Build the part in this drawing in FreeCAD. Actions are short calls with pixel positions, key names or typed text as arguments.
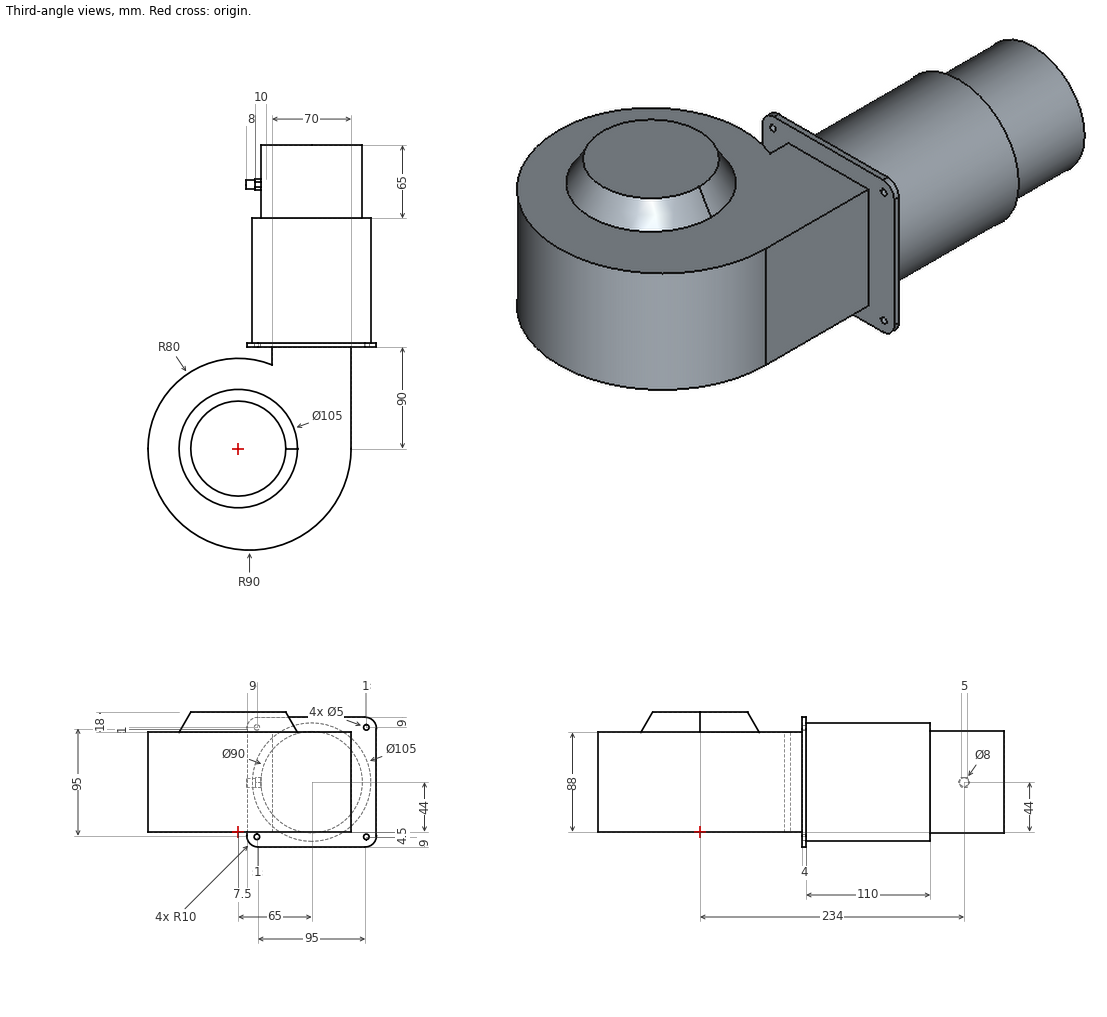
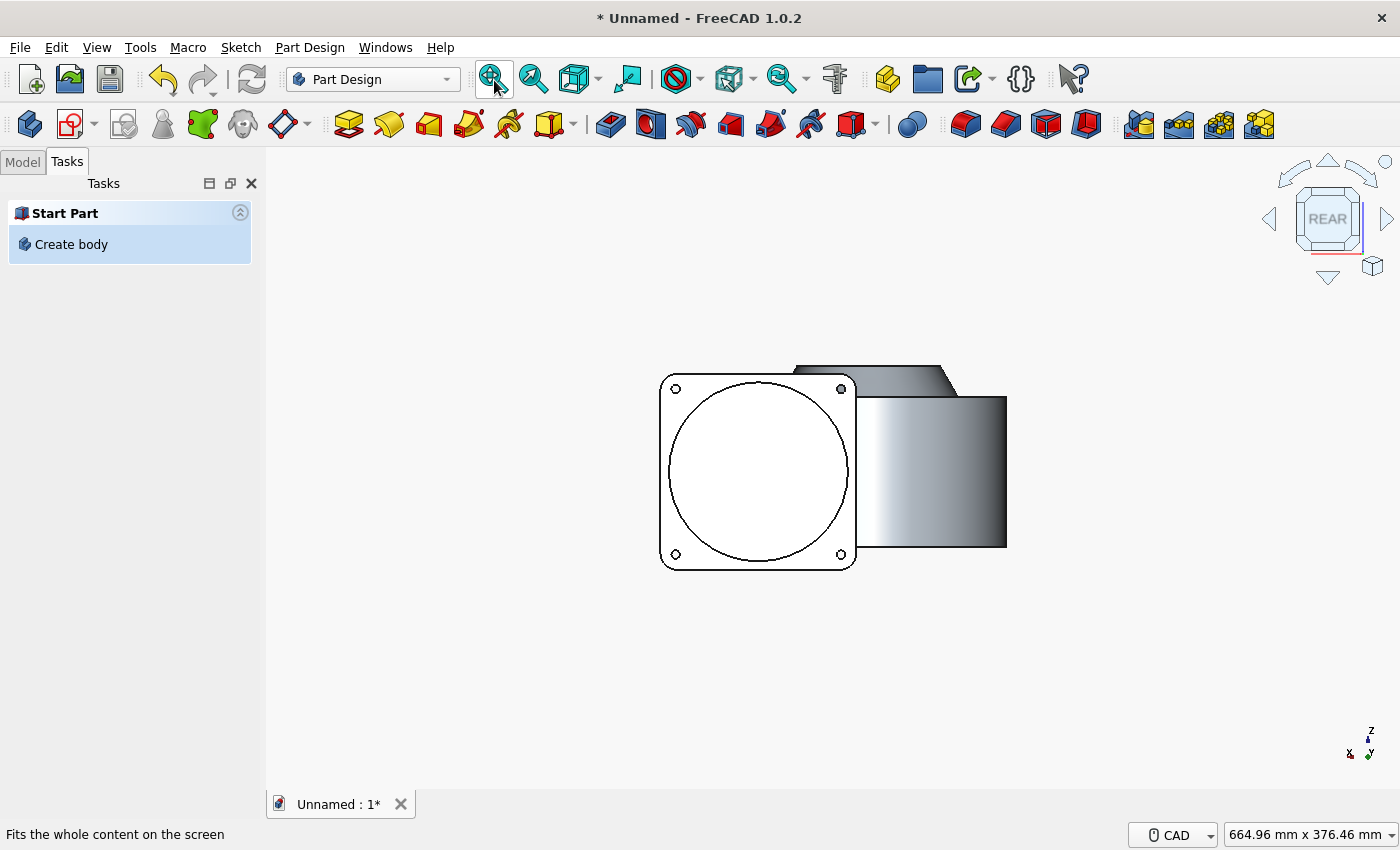
click(758, 471)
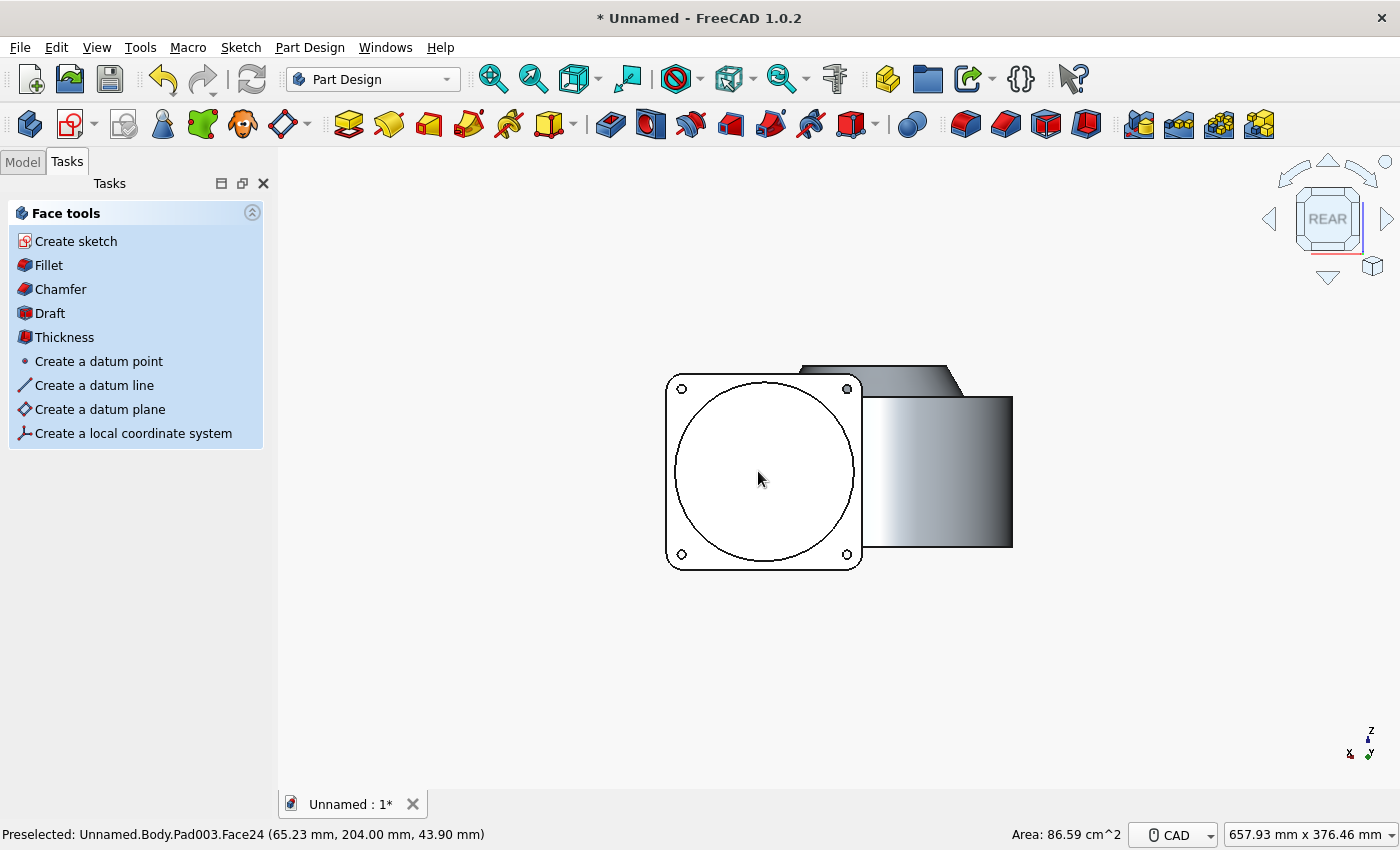
click(70, 124)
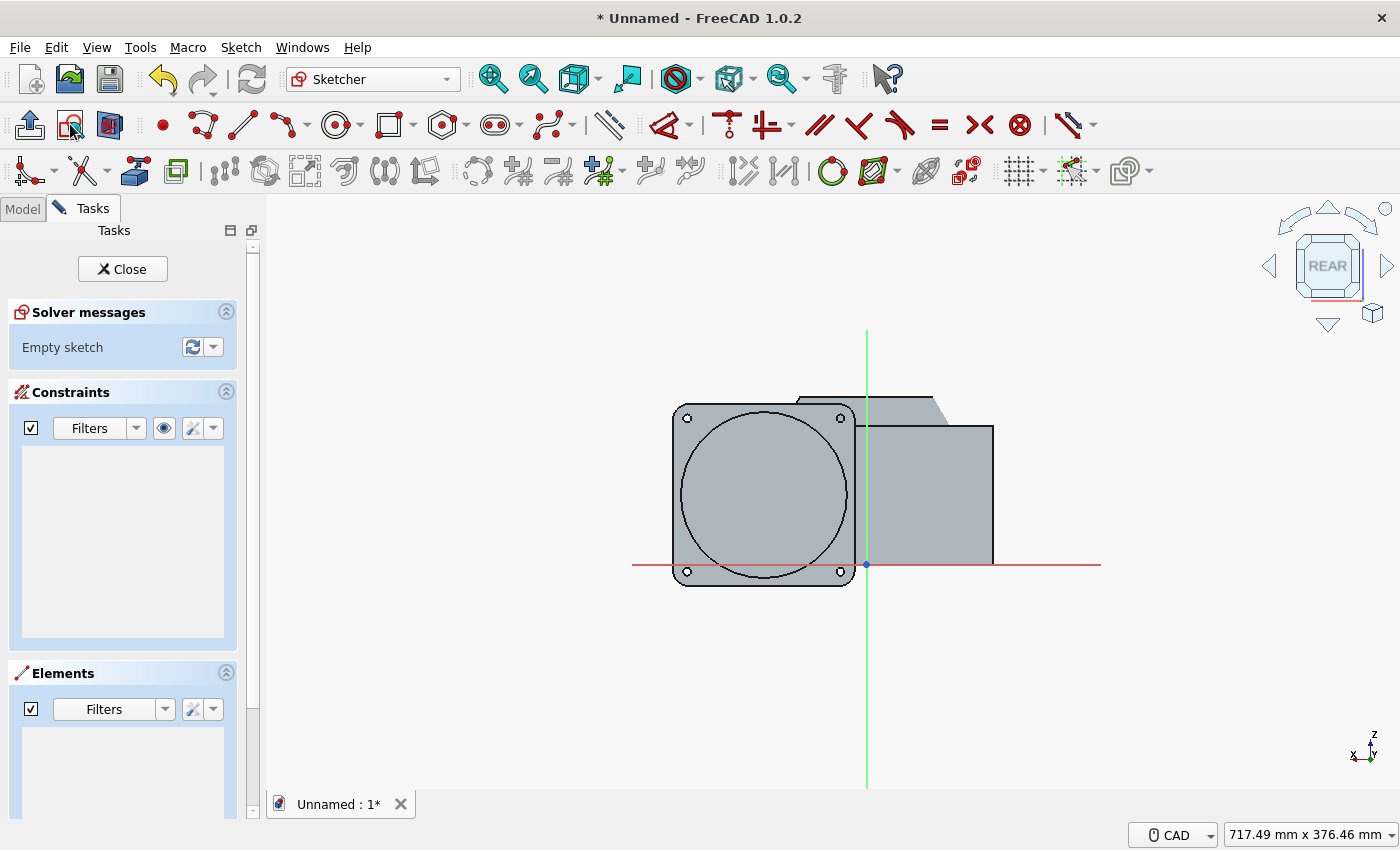
scroll(788, 497, up, 5)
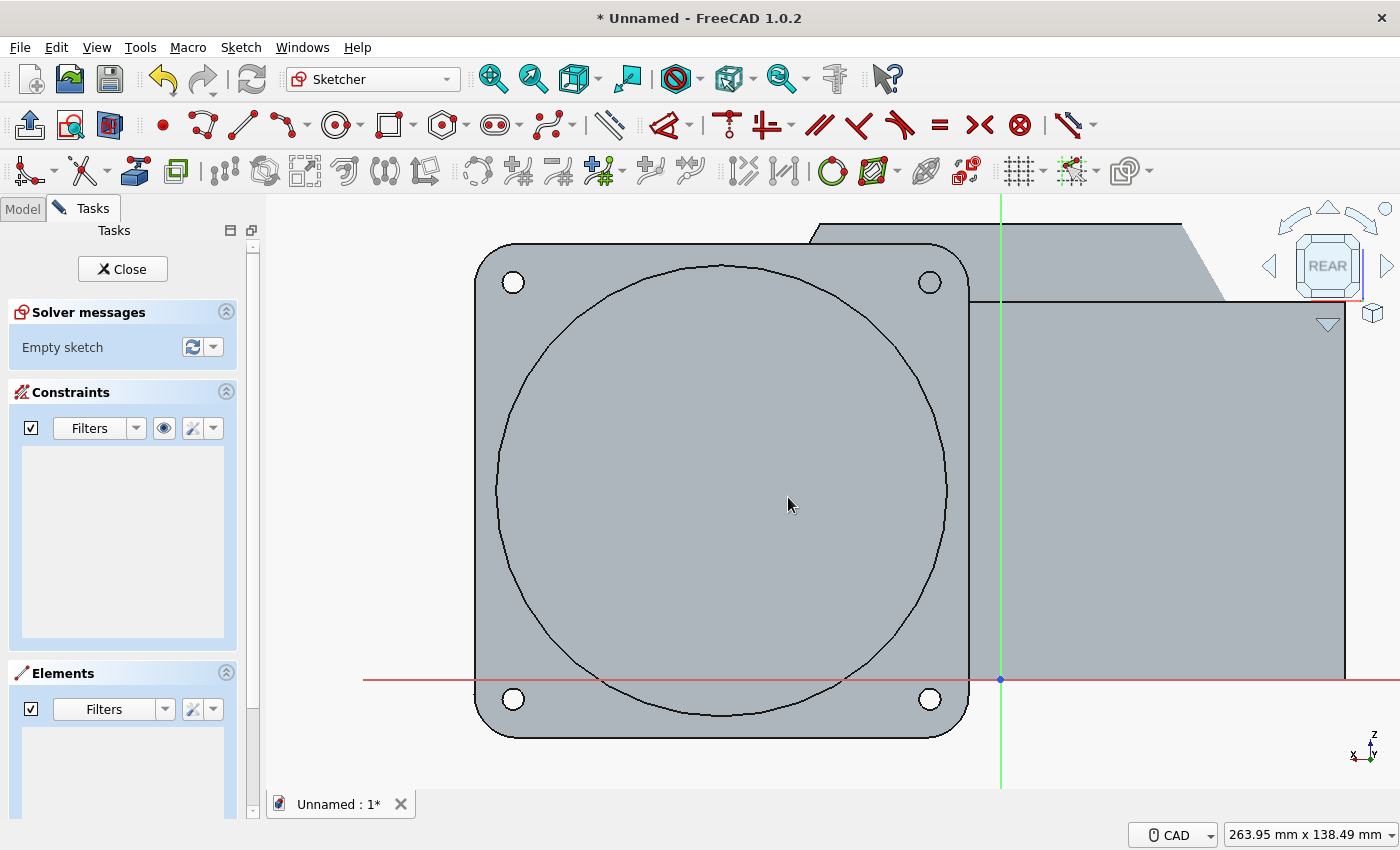
click(336, 126)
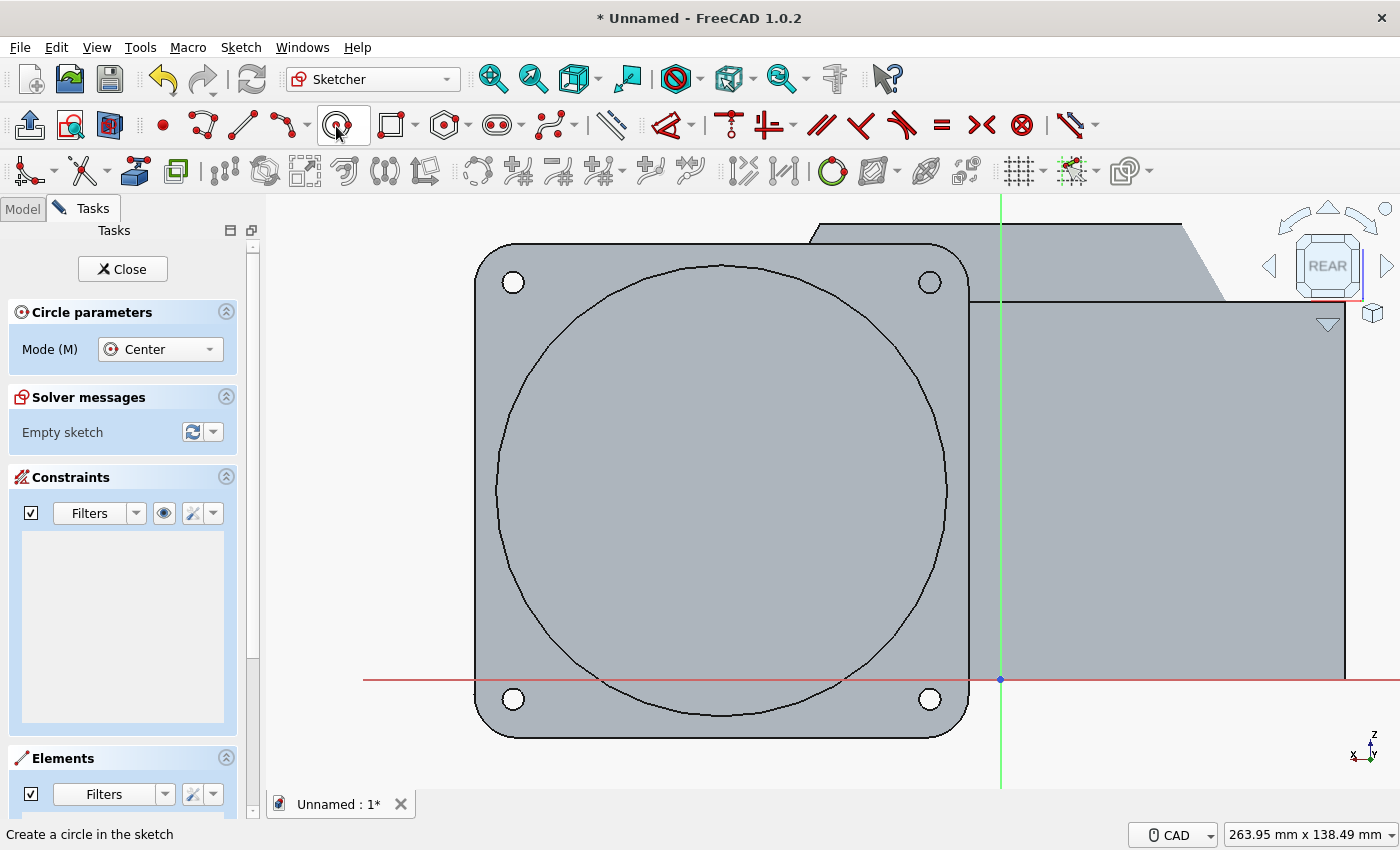
click(722, 491)
click(858, 354)
key(Escape)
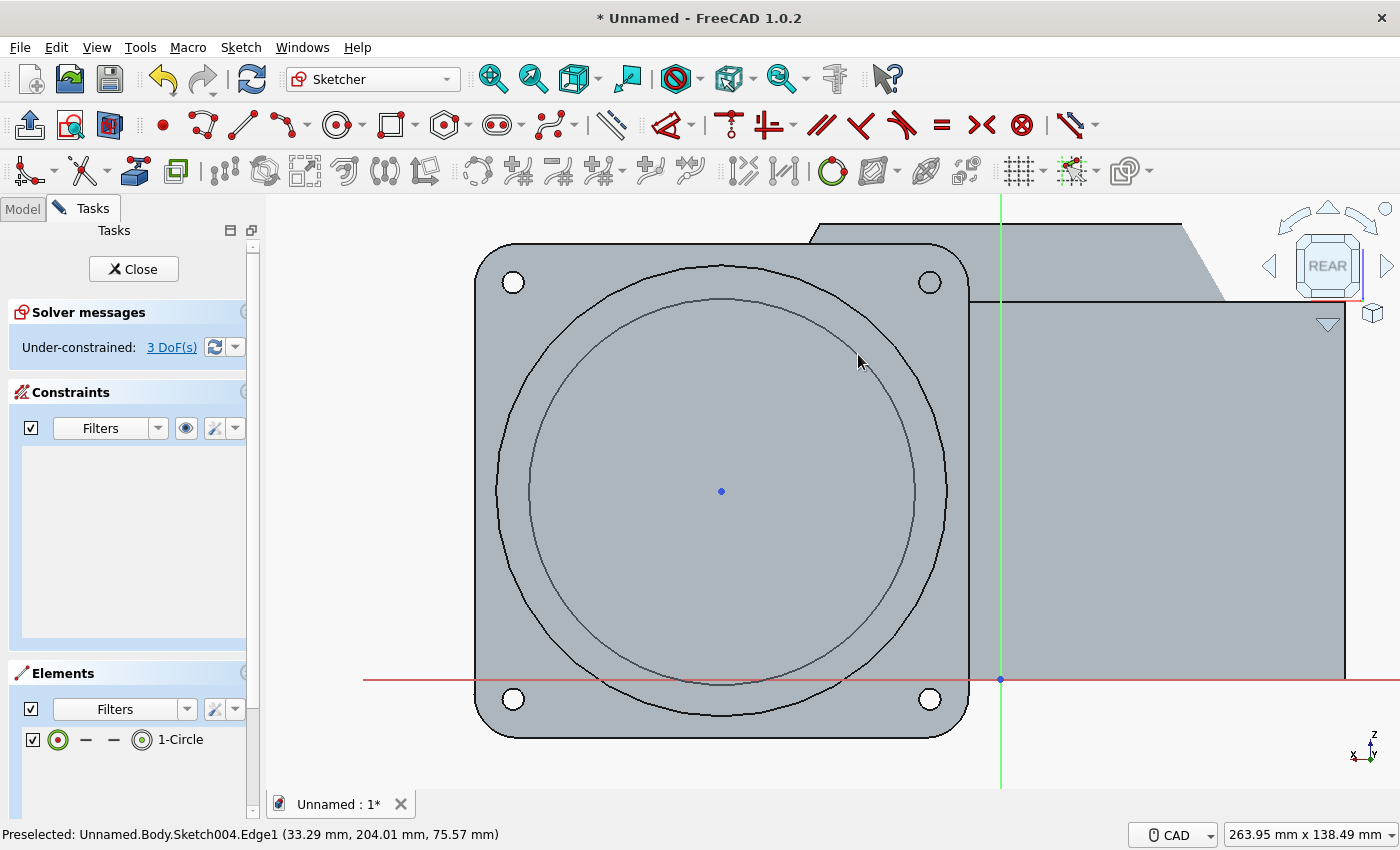
click(666, 126)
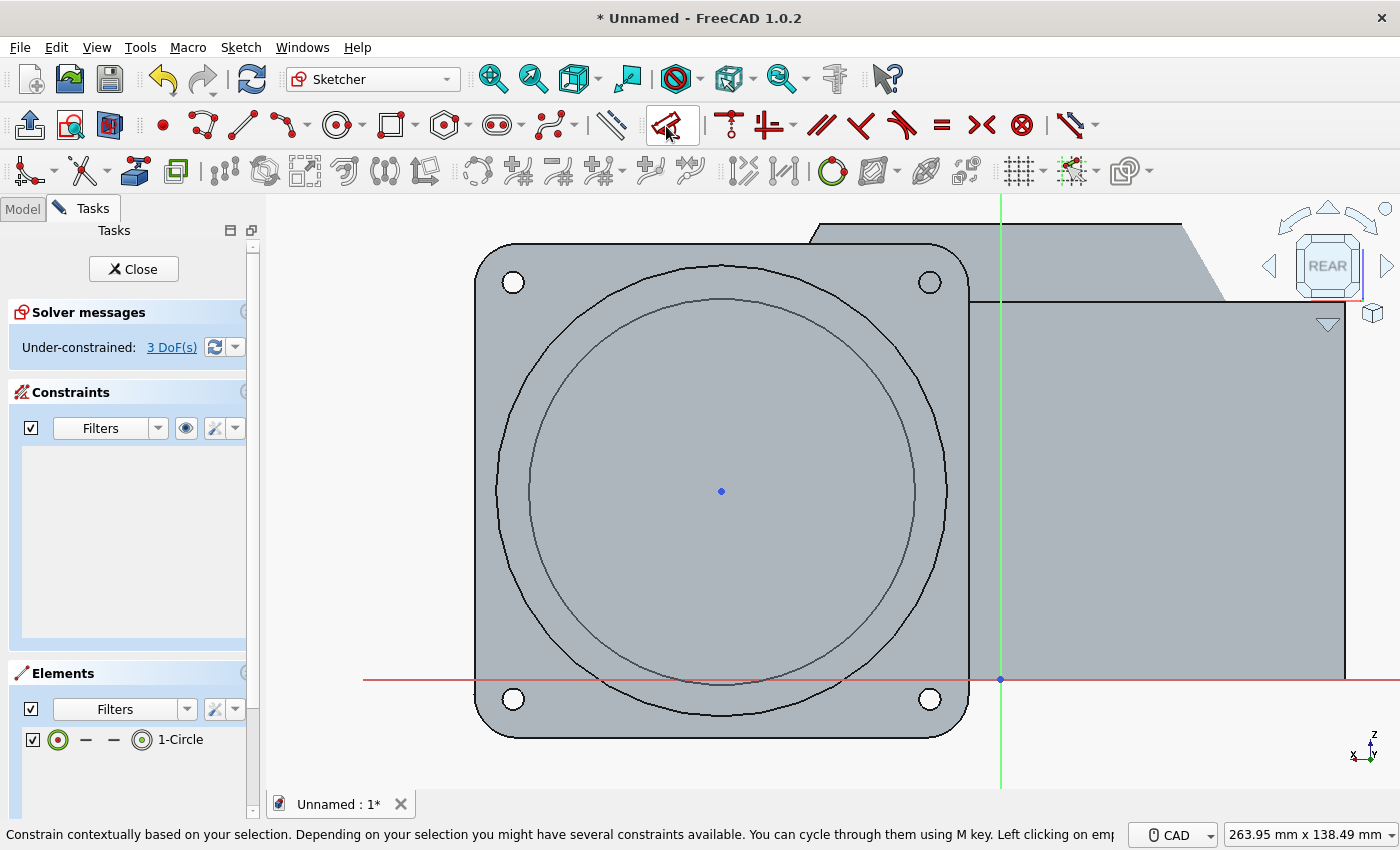
click(858, 355)
click(881, 332)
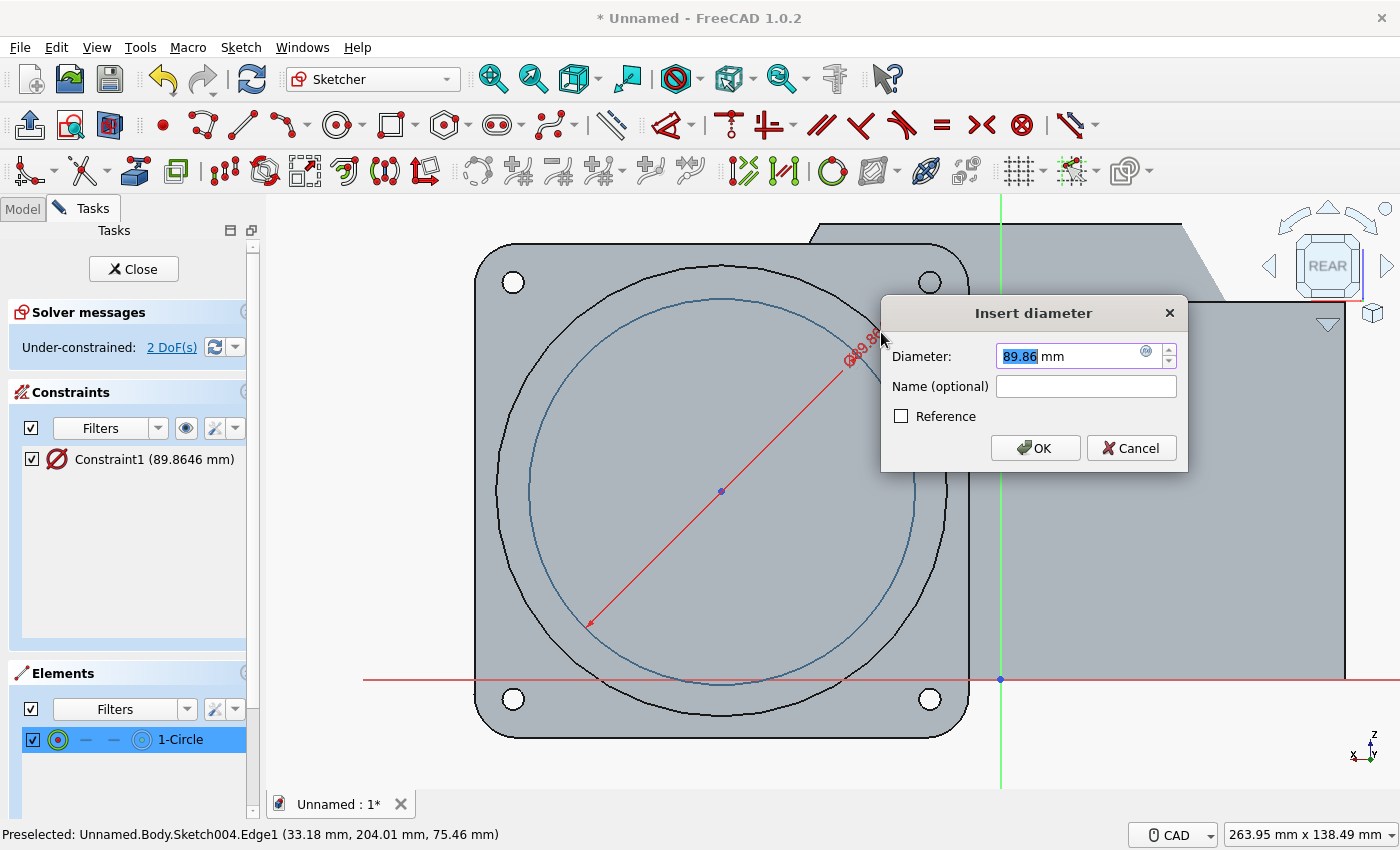
text(90)
key(Return)